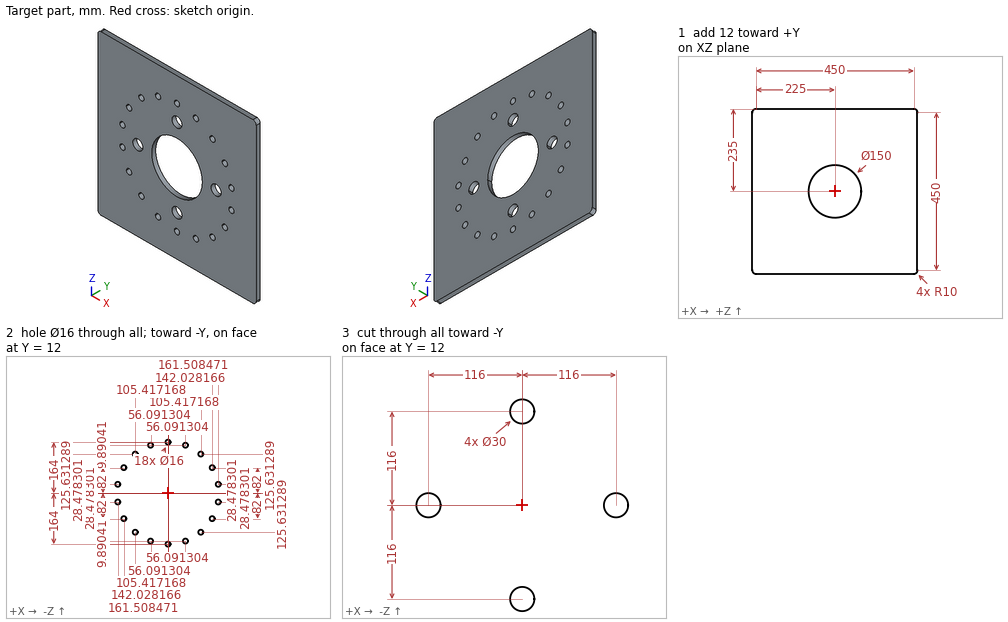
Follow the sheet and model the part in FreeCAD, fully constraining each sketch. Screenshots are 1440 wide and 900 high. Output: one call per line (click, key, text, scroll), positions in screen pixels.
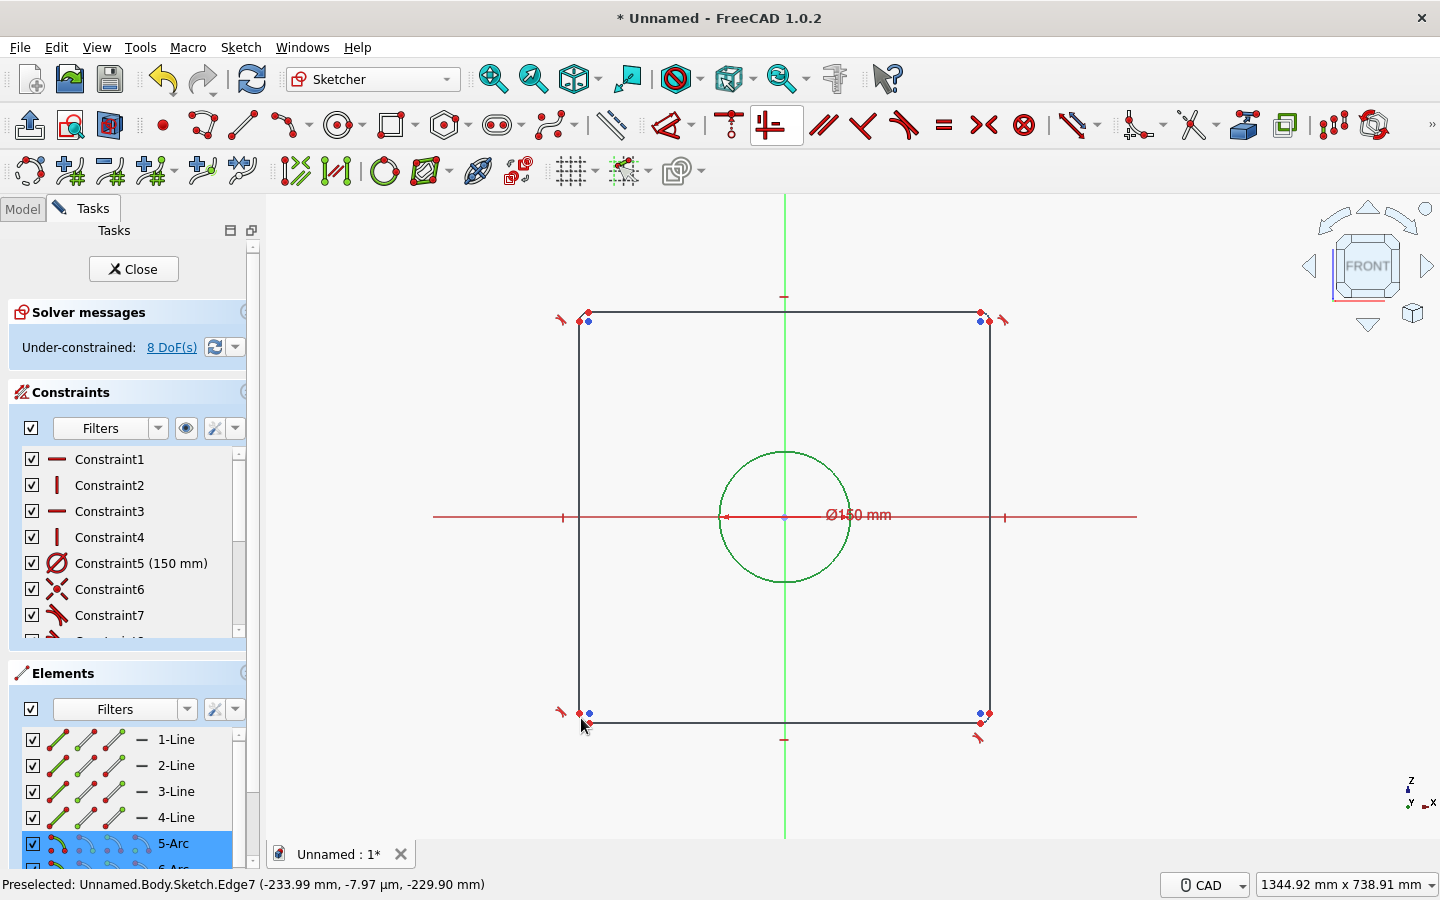
scroll(585, 313, up, 6)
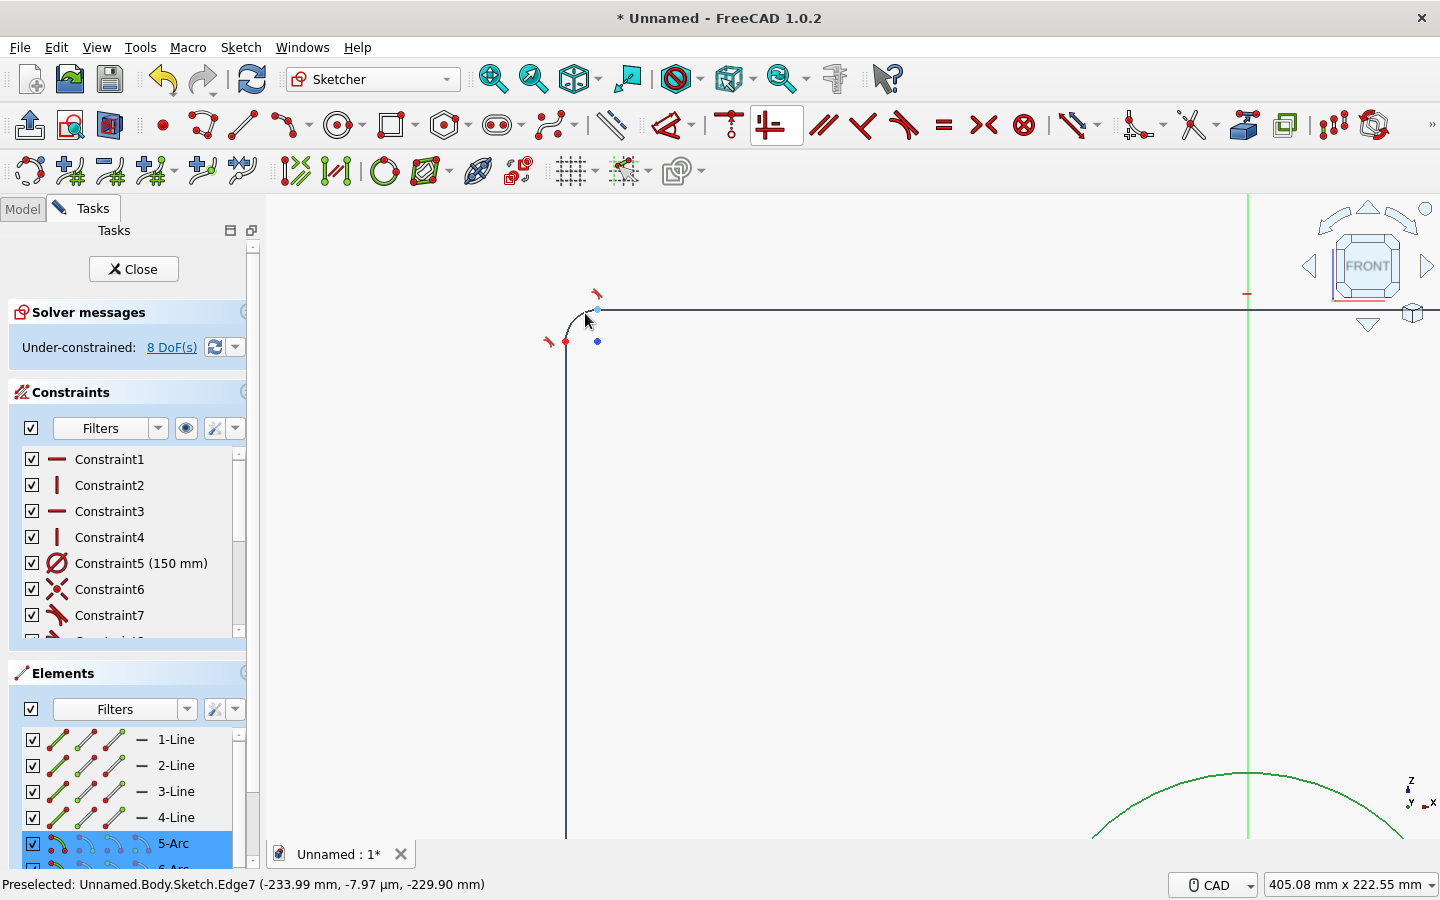
click(583, 313)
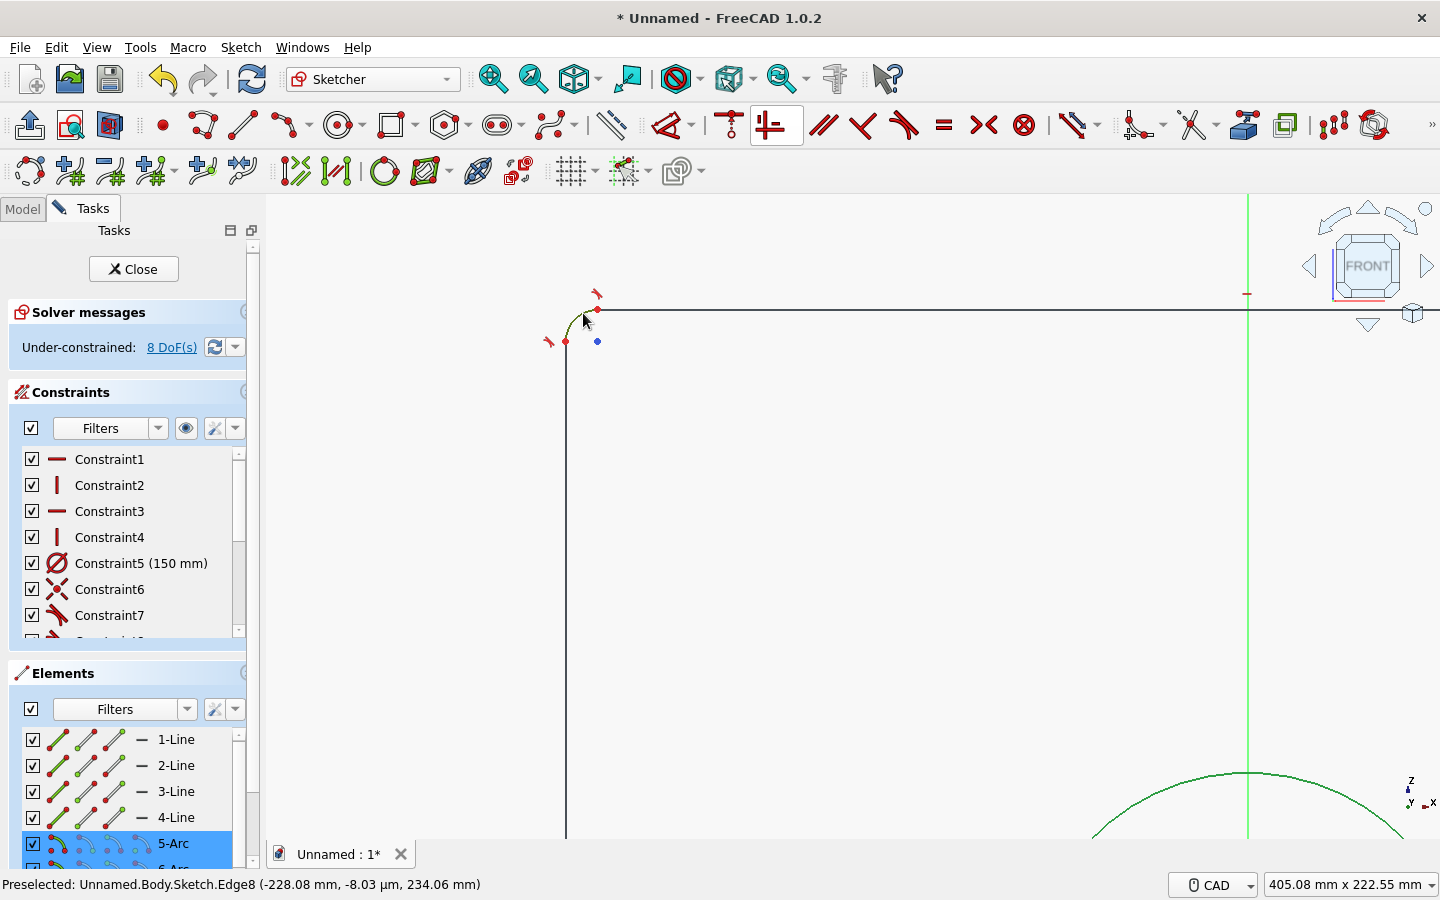
click(944, 126)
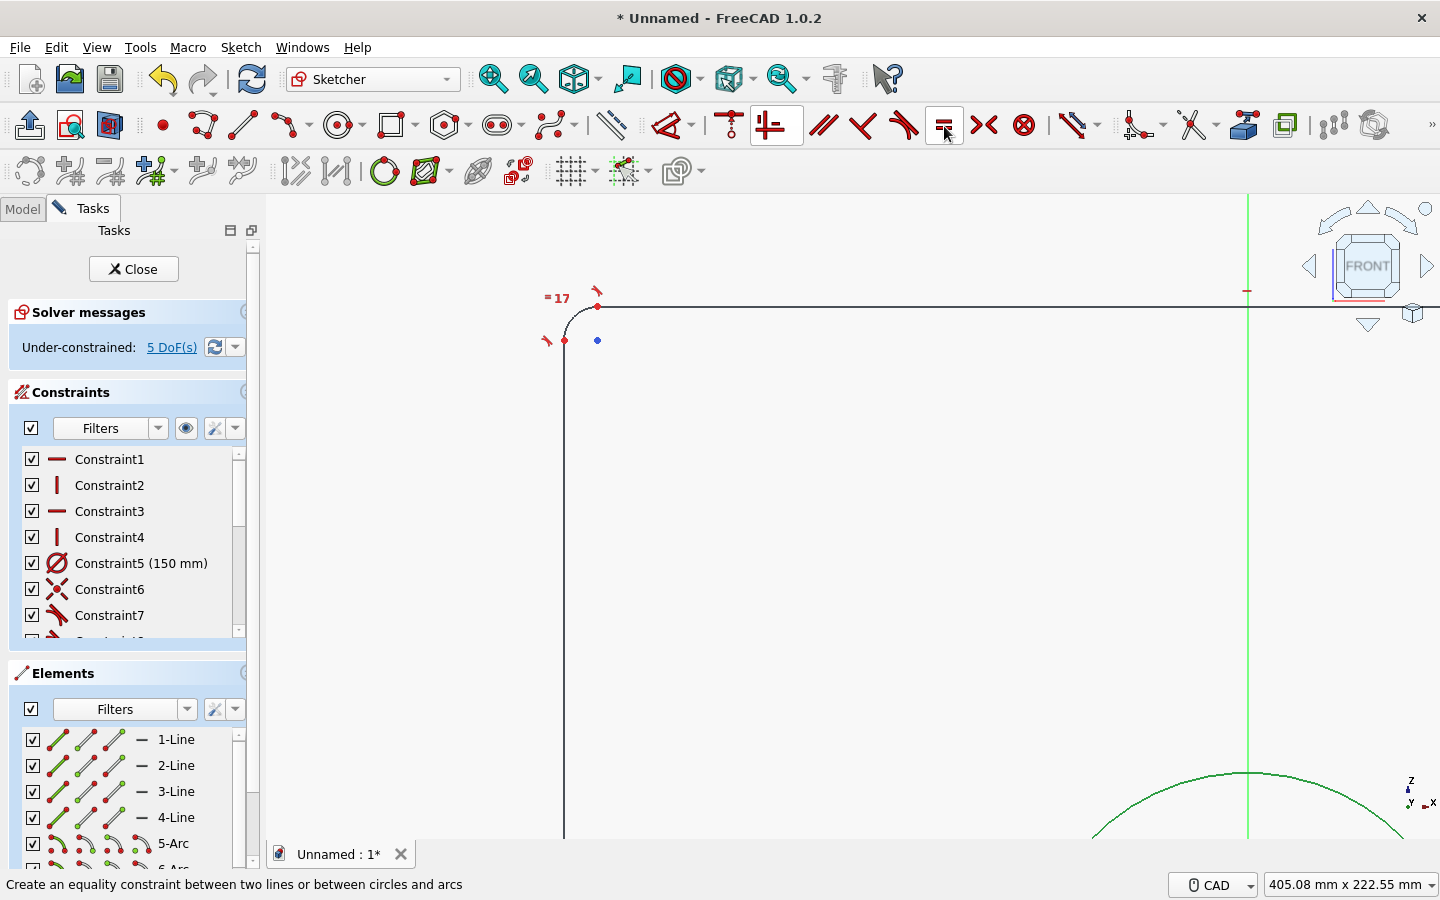
click(666, 126)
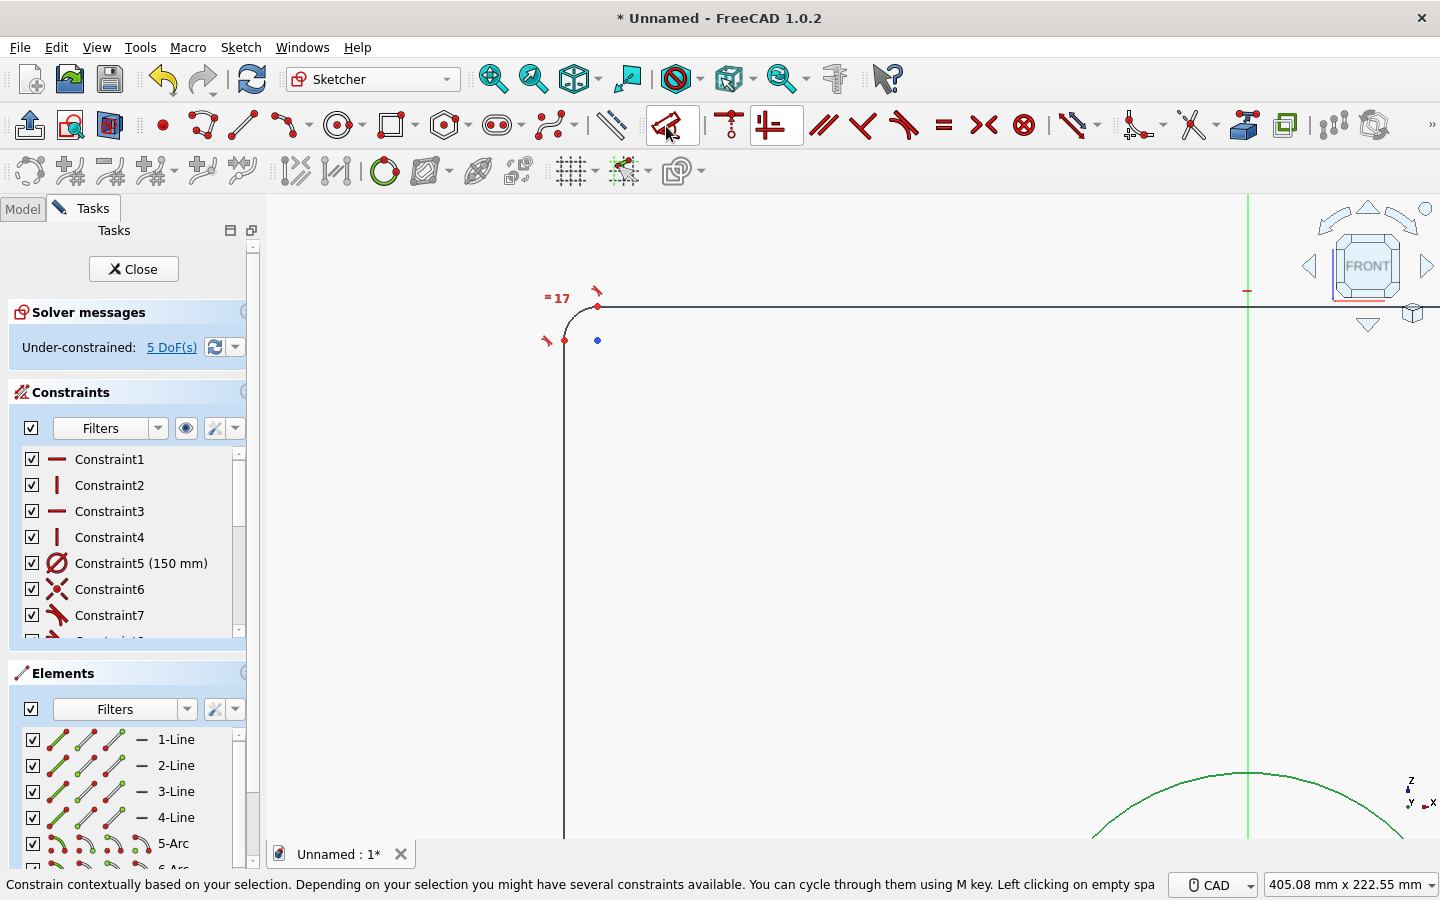
scroll(585, 312, down, 6)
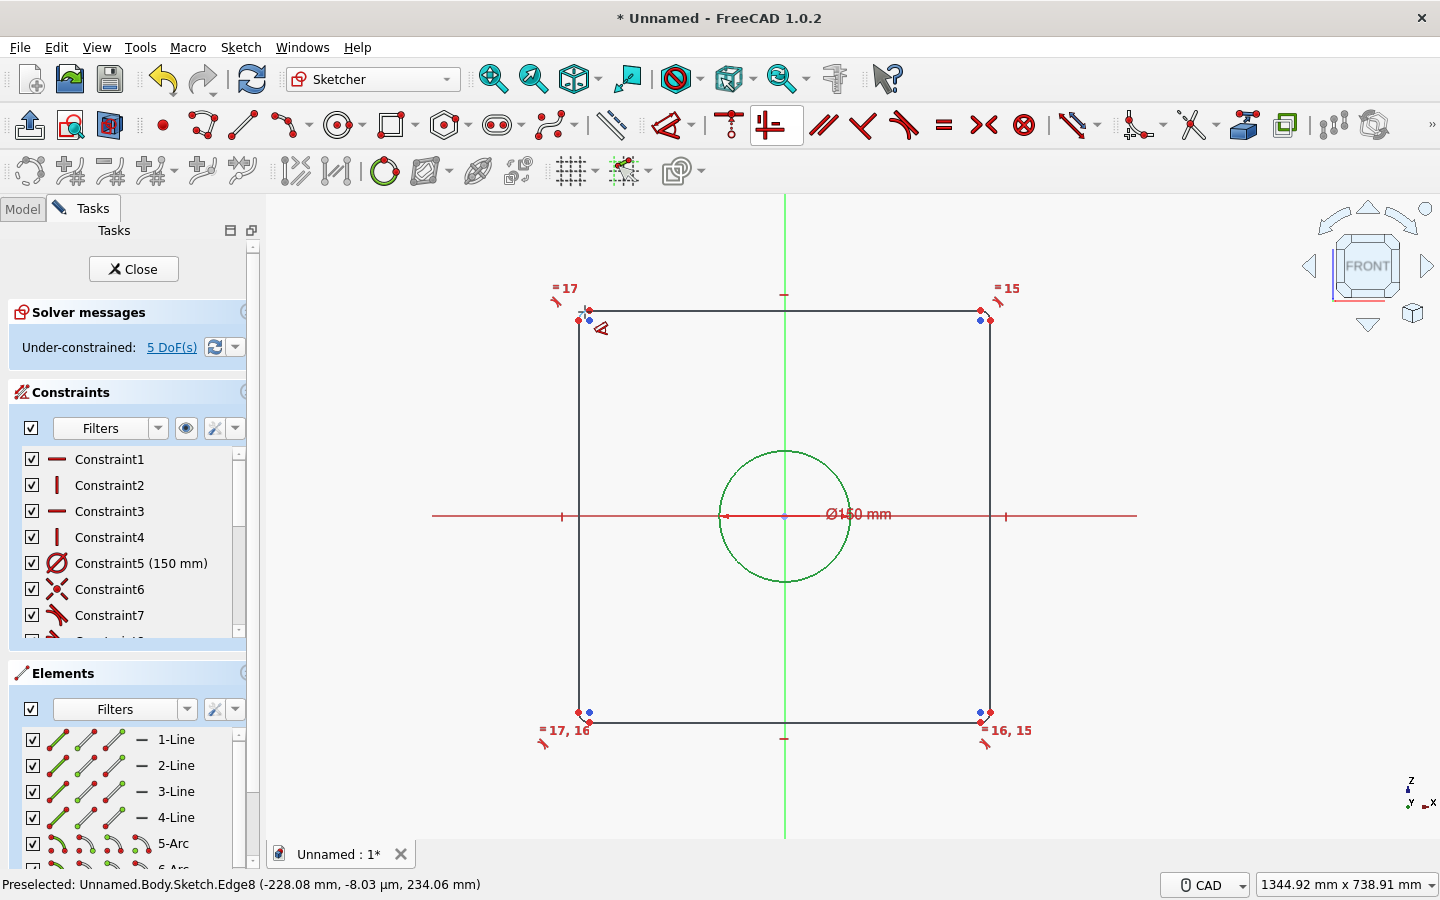
scroll(989, 316, up, 8)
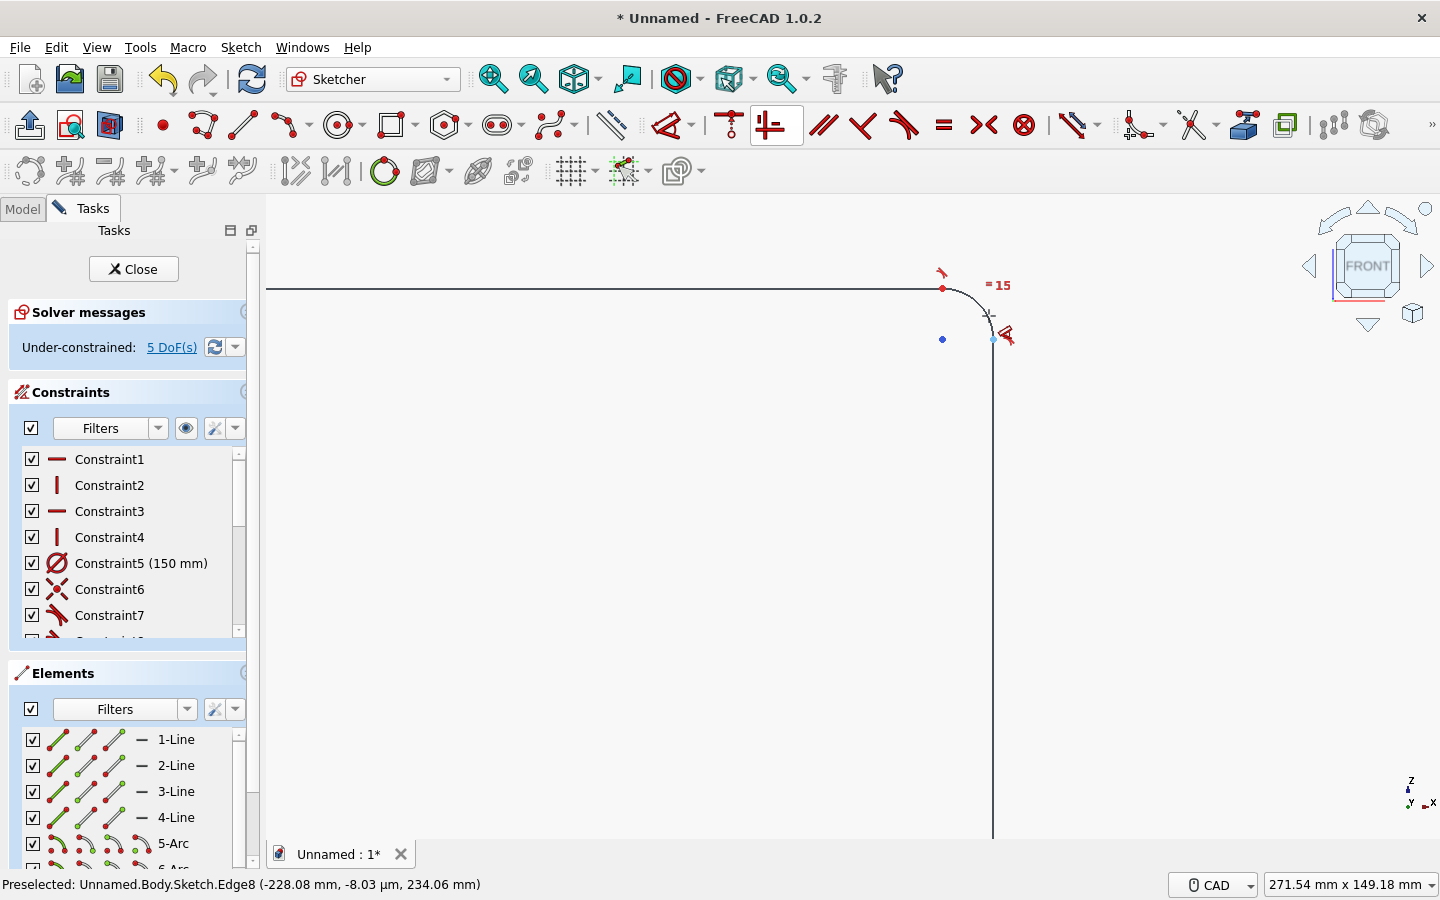
click(988, 316)
click(1016, 301)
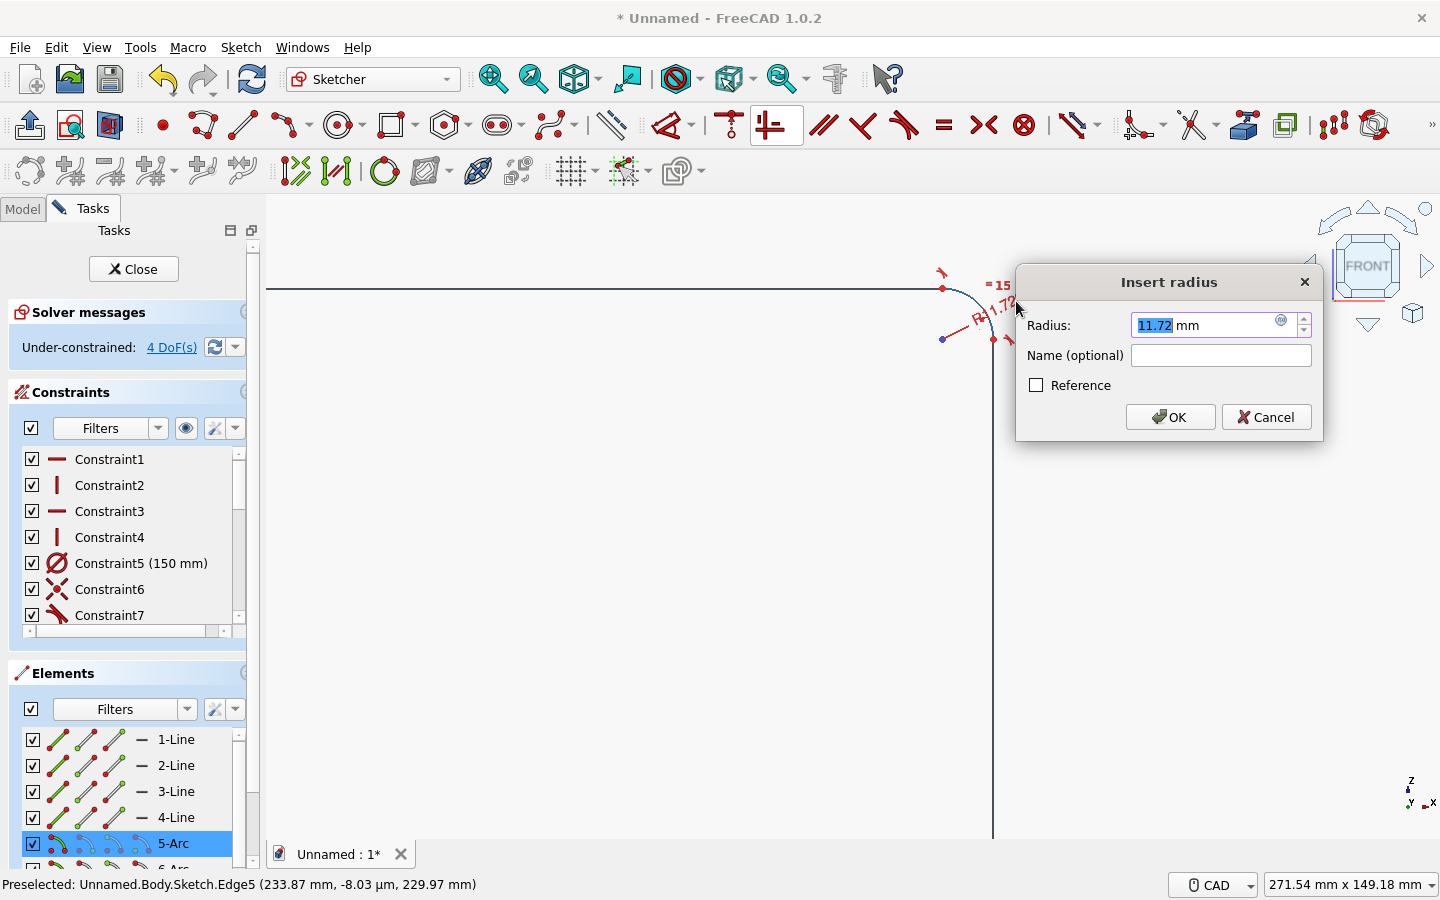
text(10)
key(Return)